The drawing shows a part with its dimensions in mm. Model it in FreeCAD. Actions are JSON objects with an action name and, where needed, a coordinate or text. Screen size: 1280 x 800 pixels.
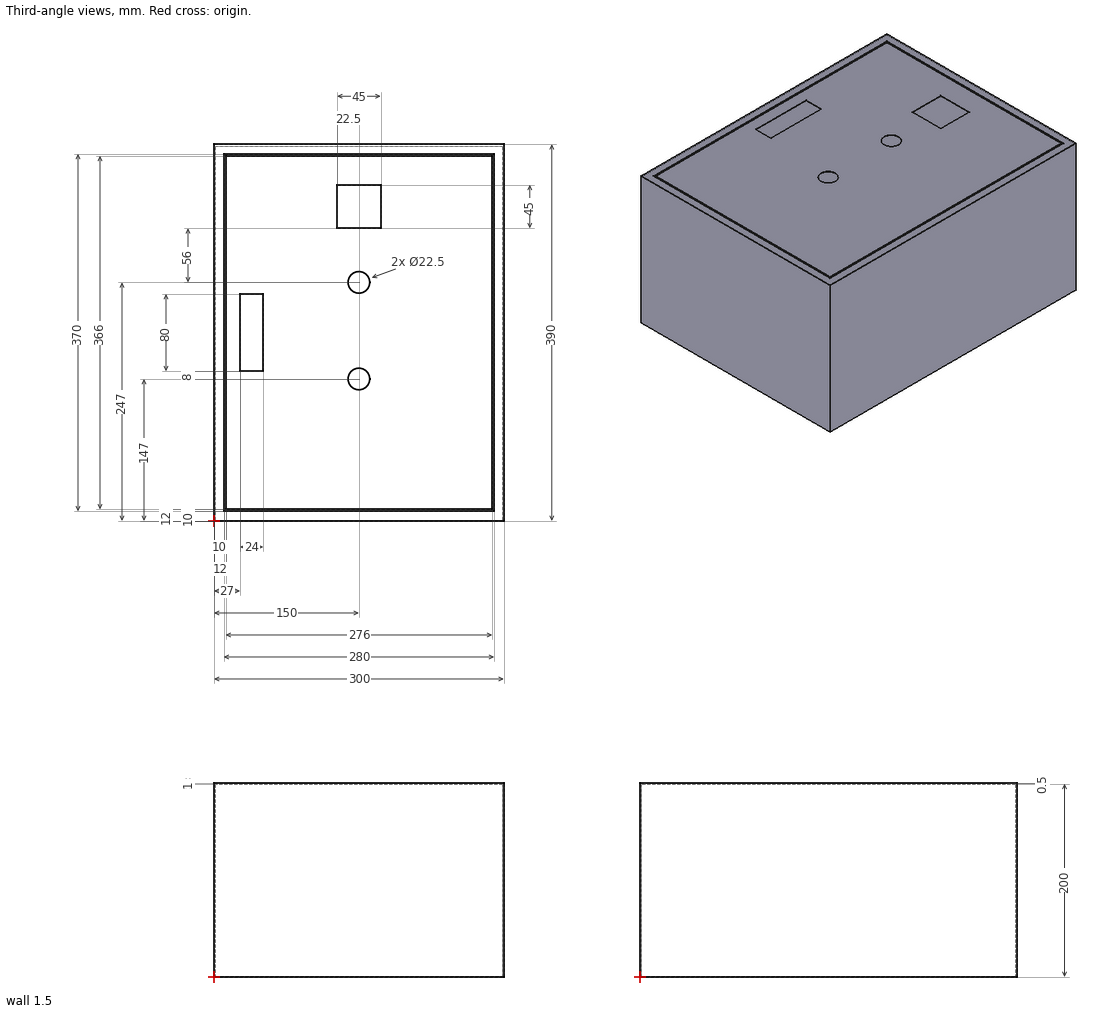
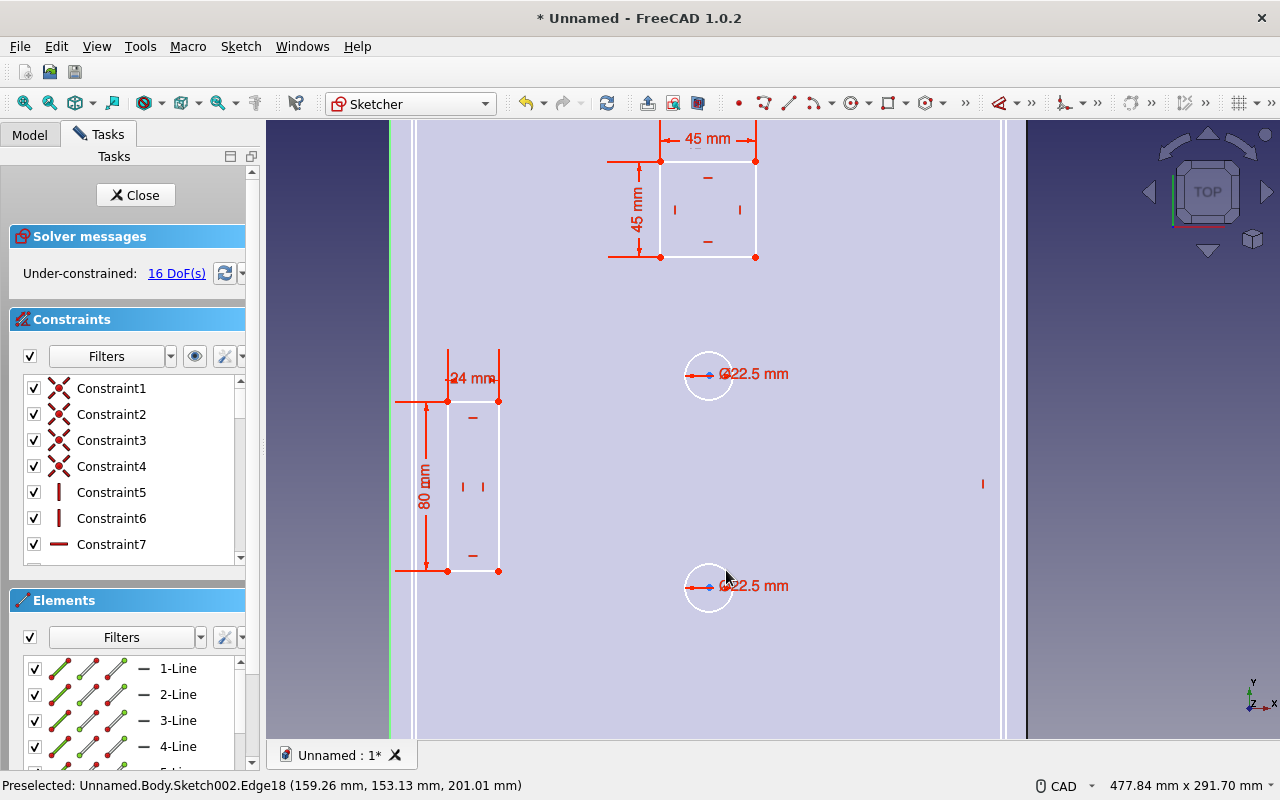
{"action": "left_click", "coordinate": [998, 104]}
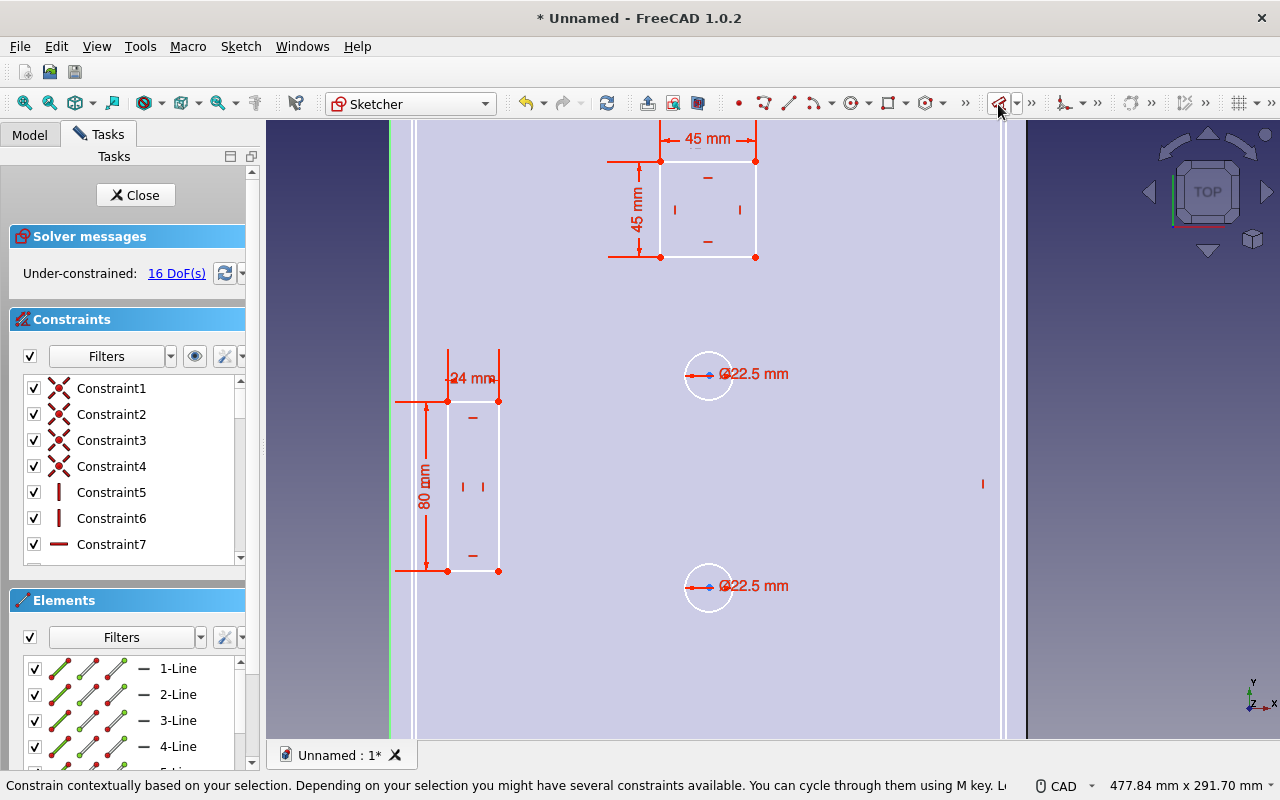
{"action": "scroll", "coordinate": [499, 571], "scroll_direction": "up", "scroll_amount": 5}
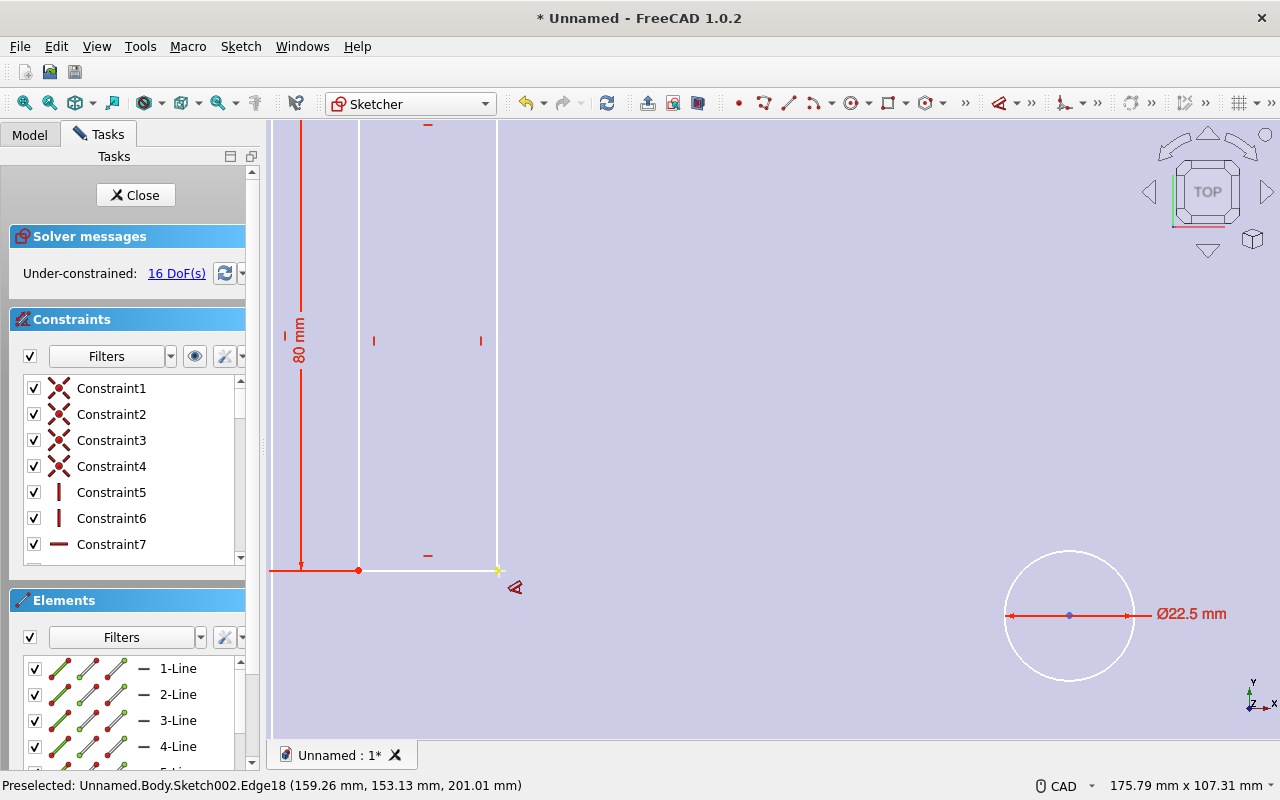
{"action": "left_click", "coordinate": [497, 571]}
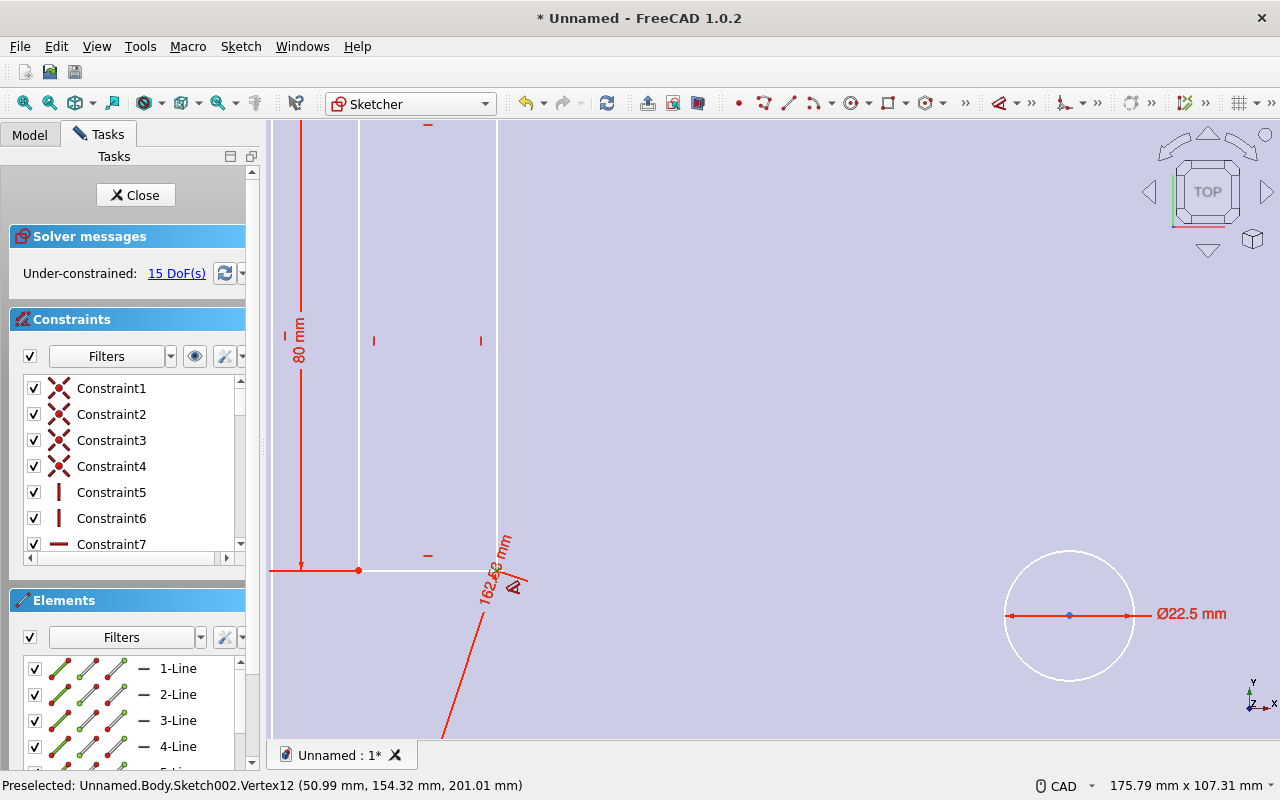
{"action": "left_click", "coordinate": [1069, 616]}
{"action": "left_click", "coordinate": [463, 593]}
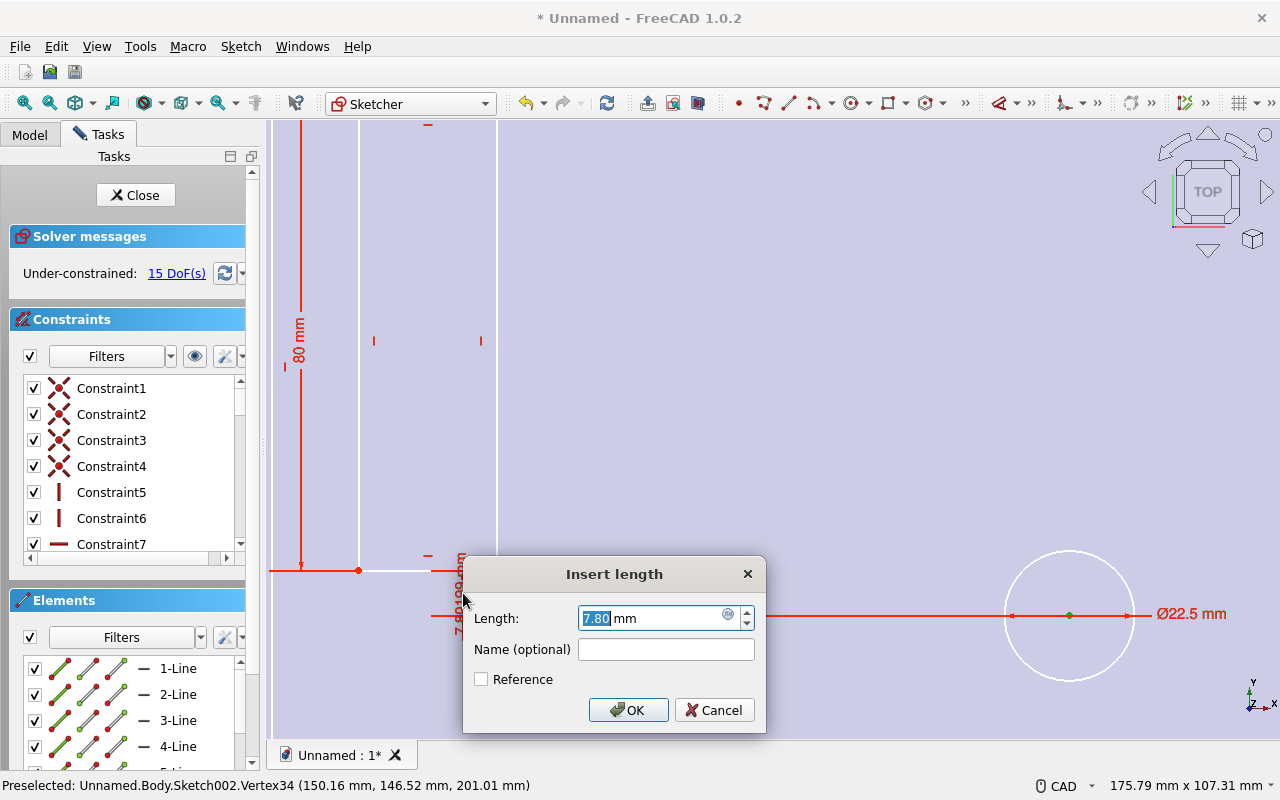
{"action": "type", "text": "8"}
{"action": "key", "text": "Return"}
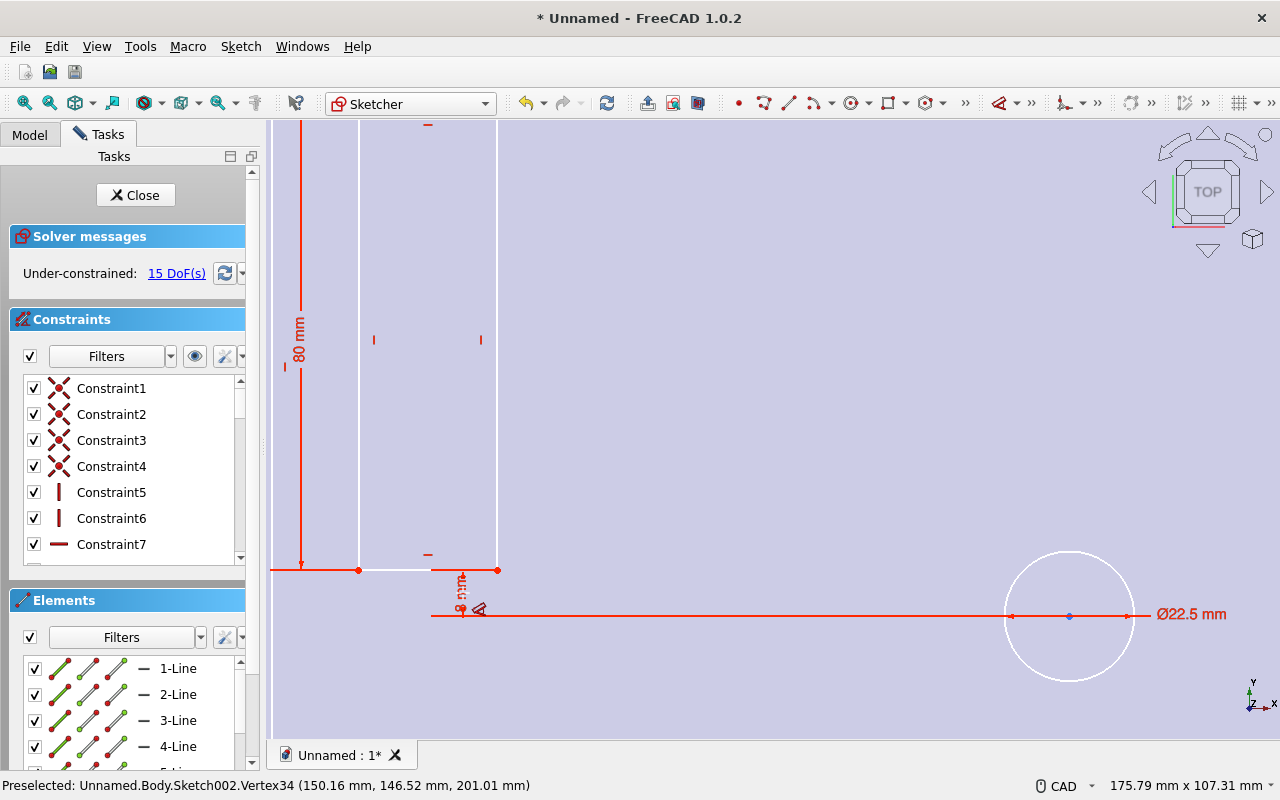
{"action": "scroll", "coordinate": [638, 442], "scroll_direction": "down", "scroll_amount": 9}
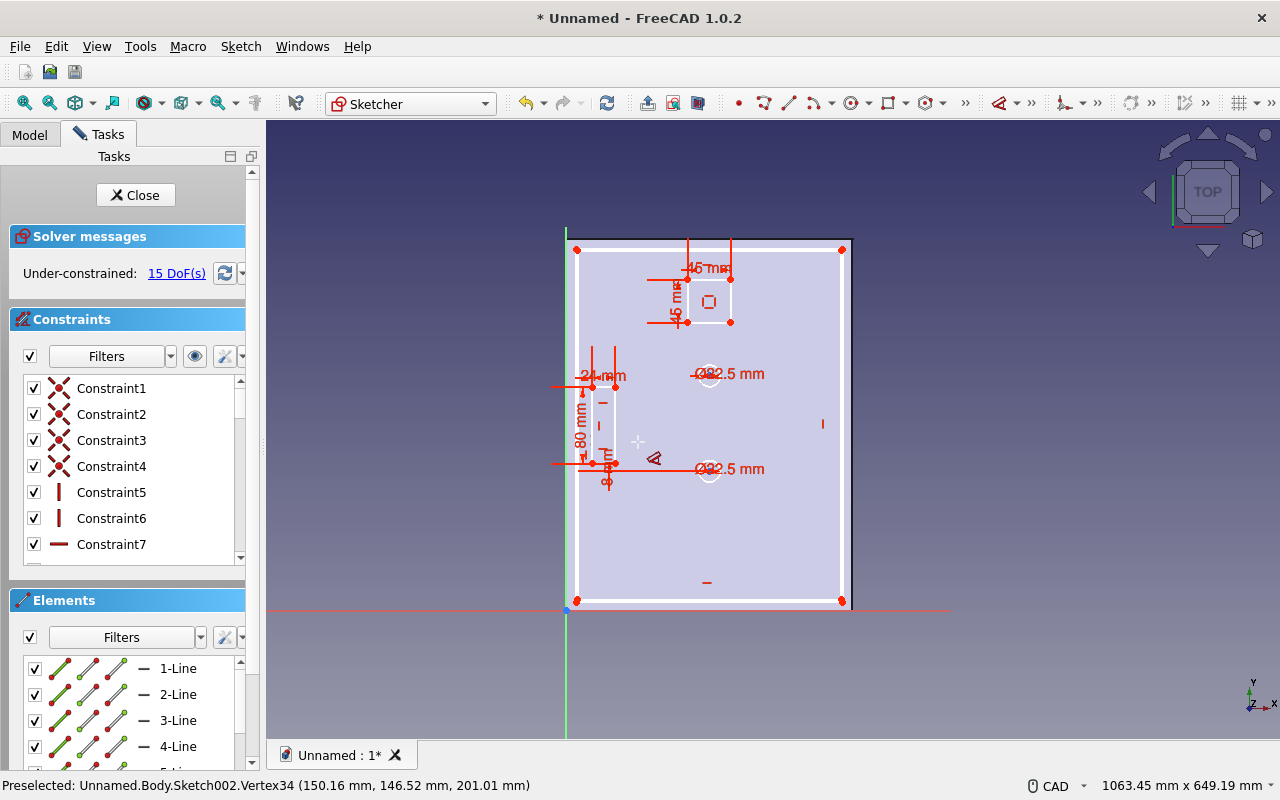
{"action": "scroll", "coordinate": [576, 355], "scroll_direction": "up", "scroll_amount": 11}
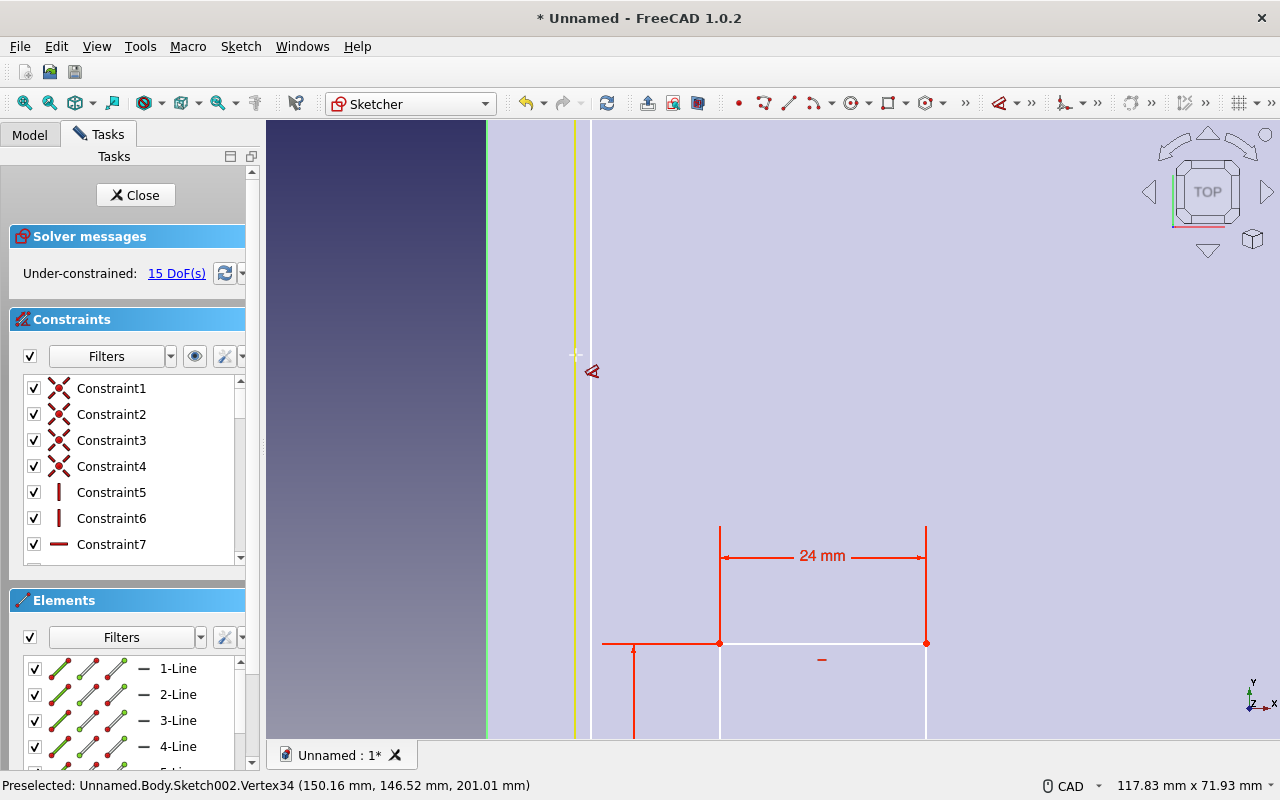
{"action": "left_click", "coordinate": [575, 352]}
{"action": "left_click", "coordinate": [541, 430]}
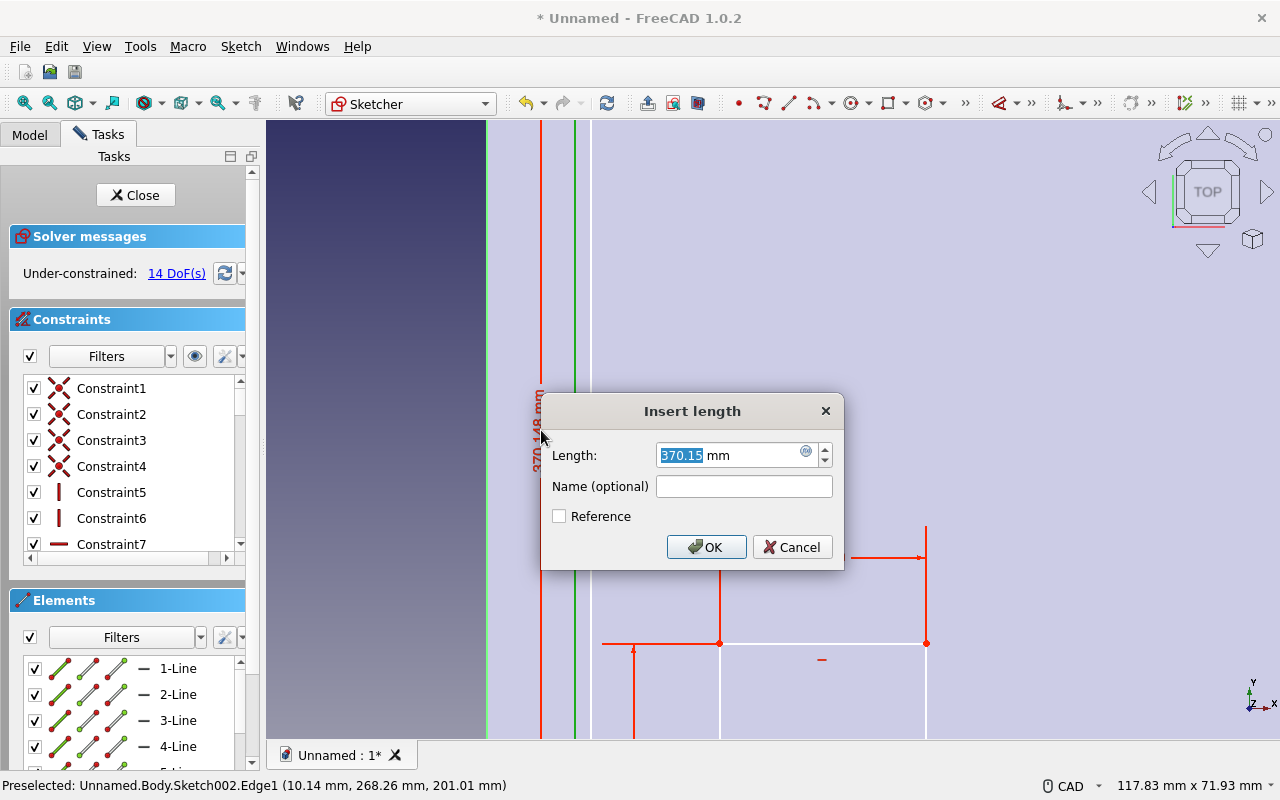
{"action": "type", "text": "370"}
{"action": "key", "text": "Return"}